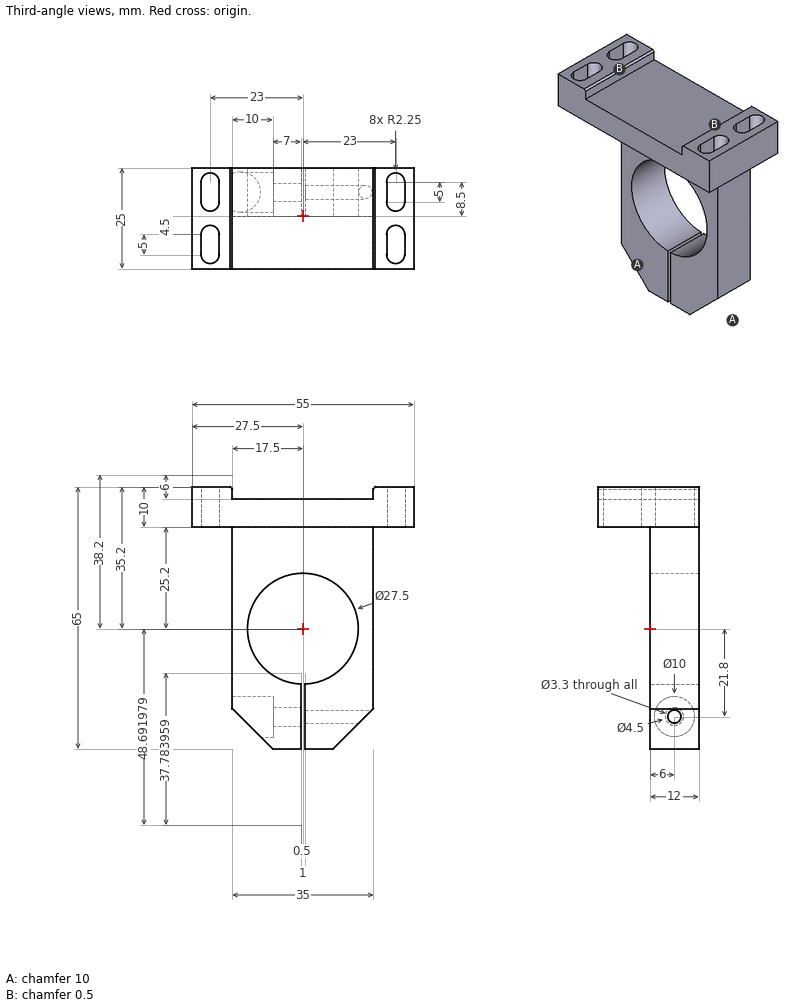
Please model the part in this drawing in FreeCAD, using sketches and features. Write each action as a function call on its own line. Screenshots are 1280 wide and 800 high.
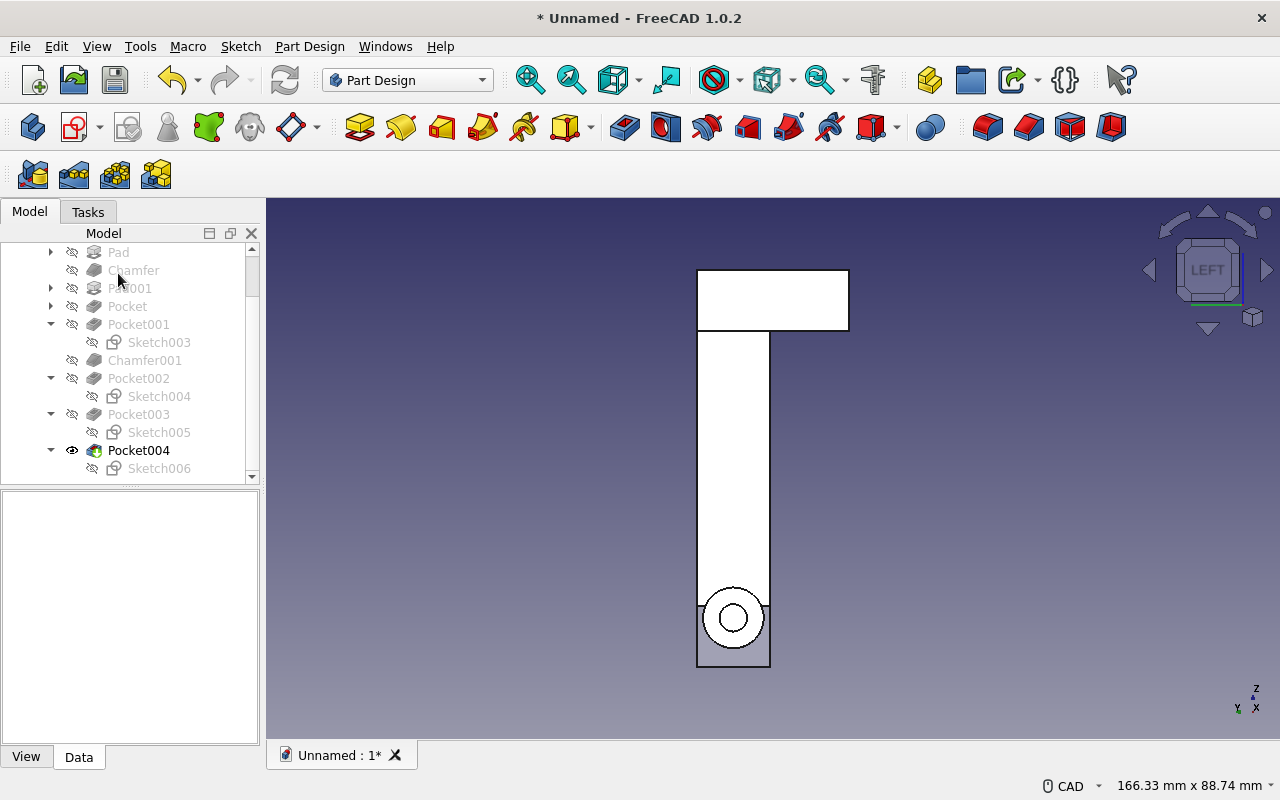
click(733, 617)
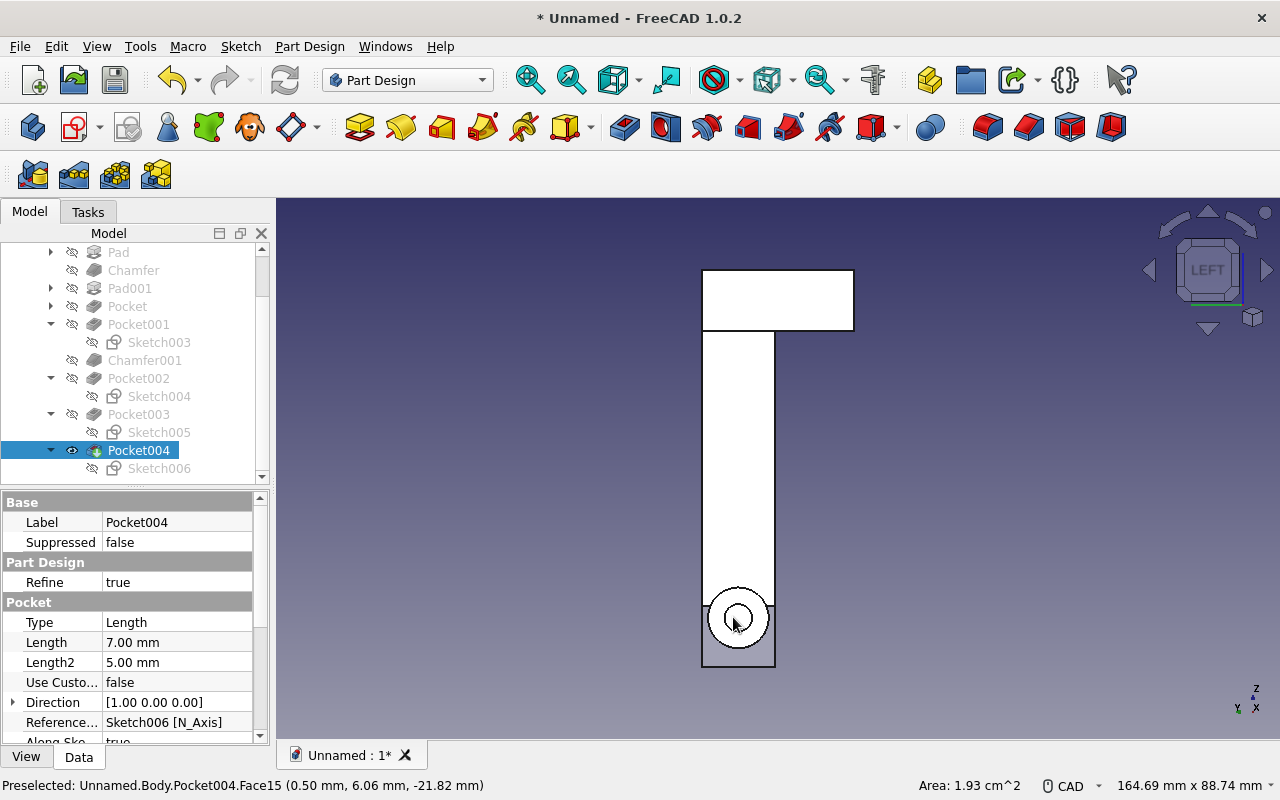
click(74, 128)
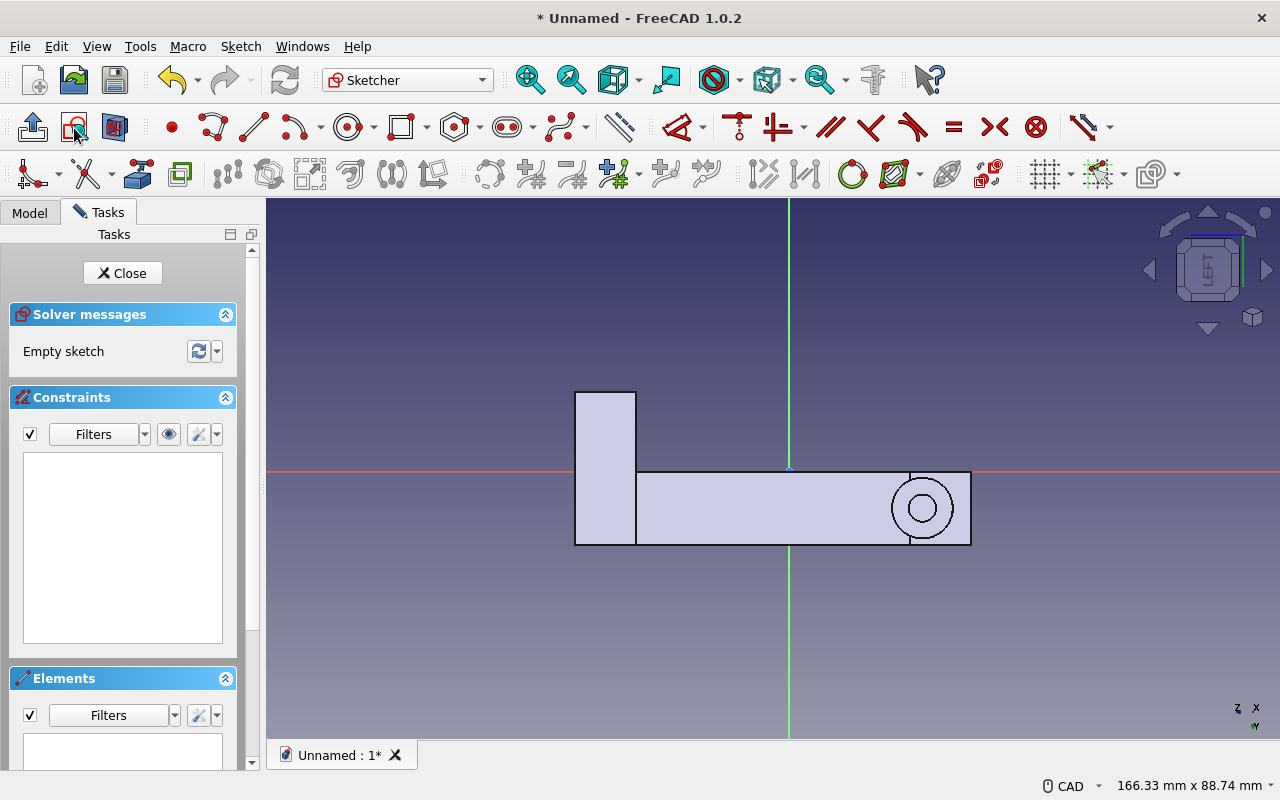
scroll(936, 511, up, 14)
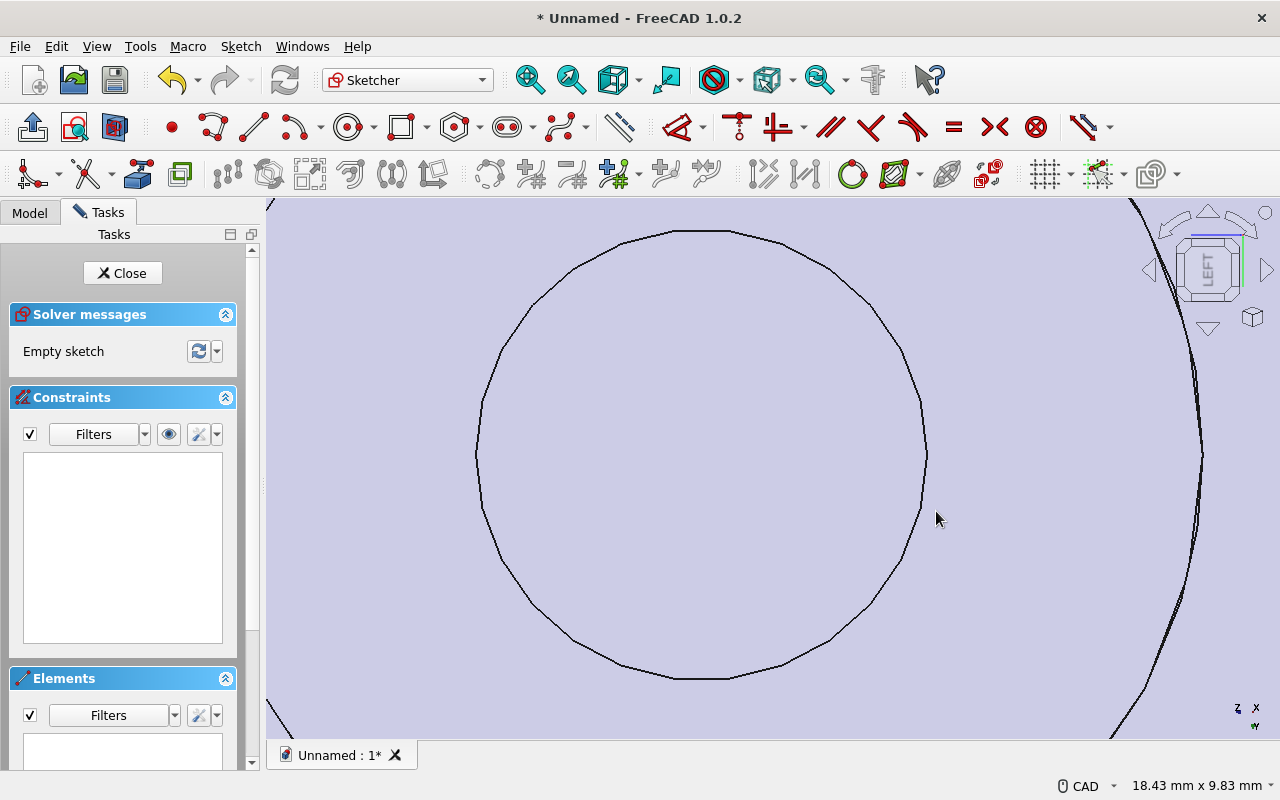
click(348, 128)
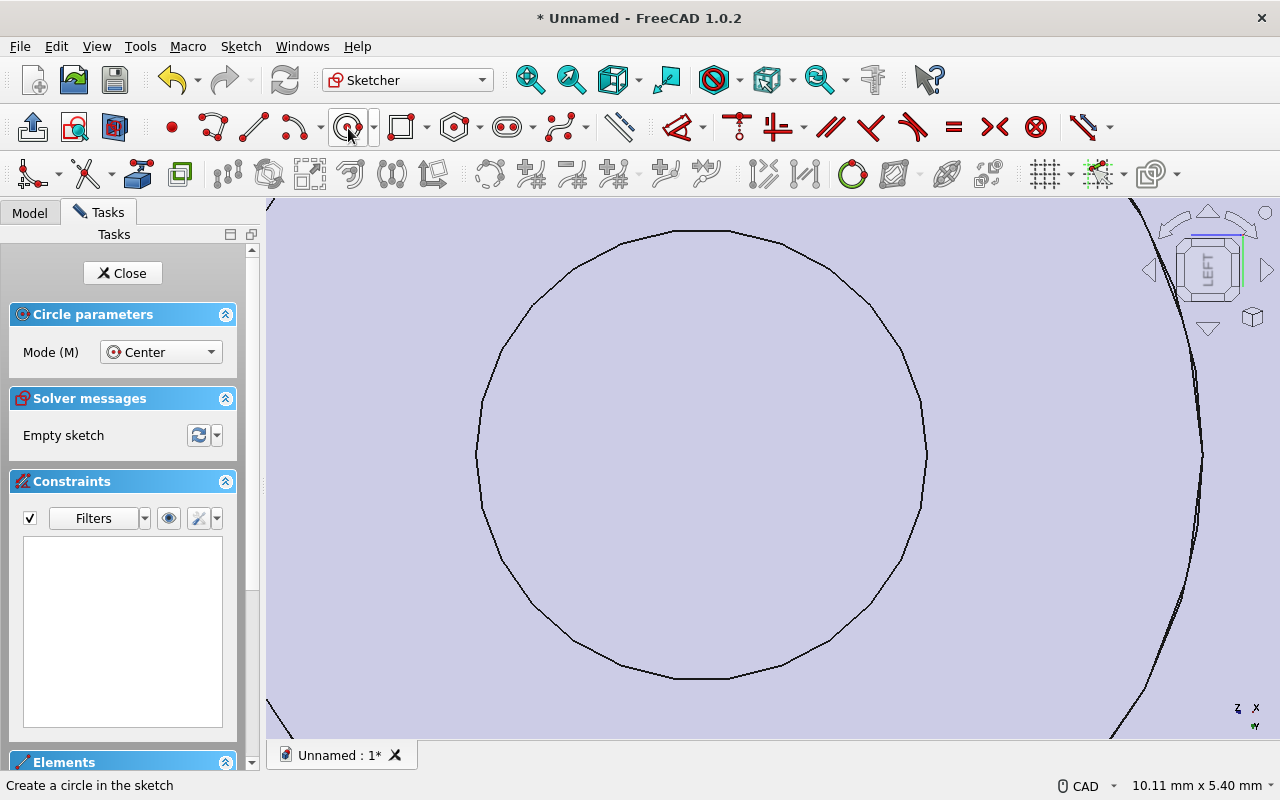
click(702, 455)
click(818, 338)
key(Escape)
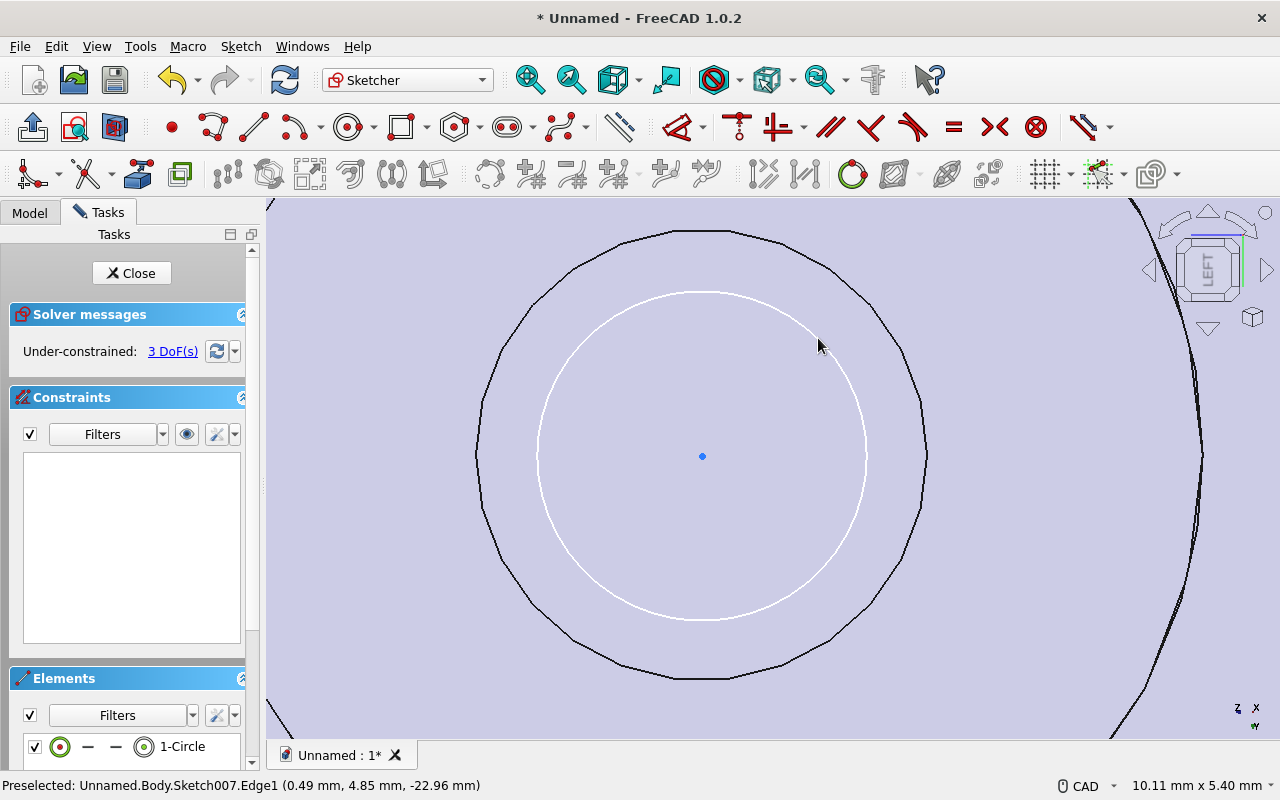
click(676, 128)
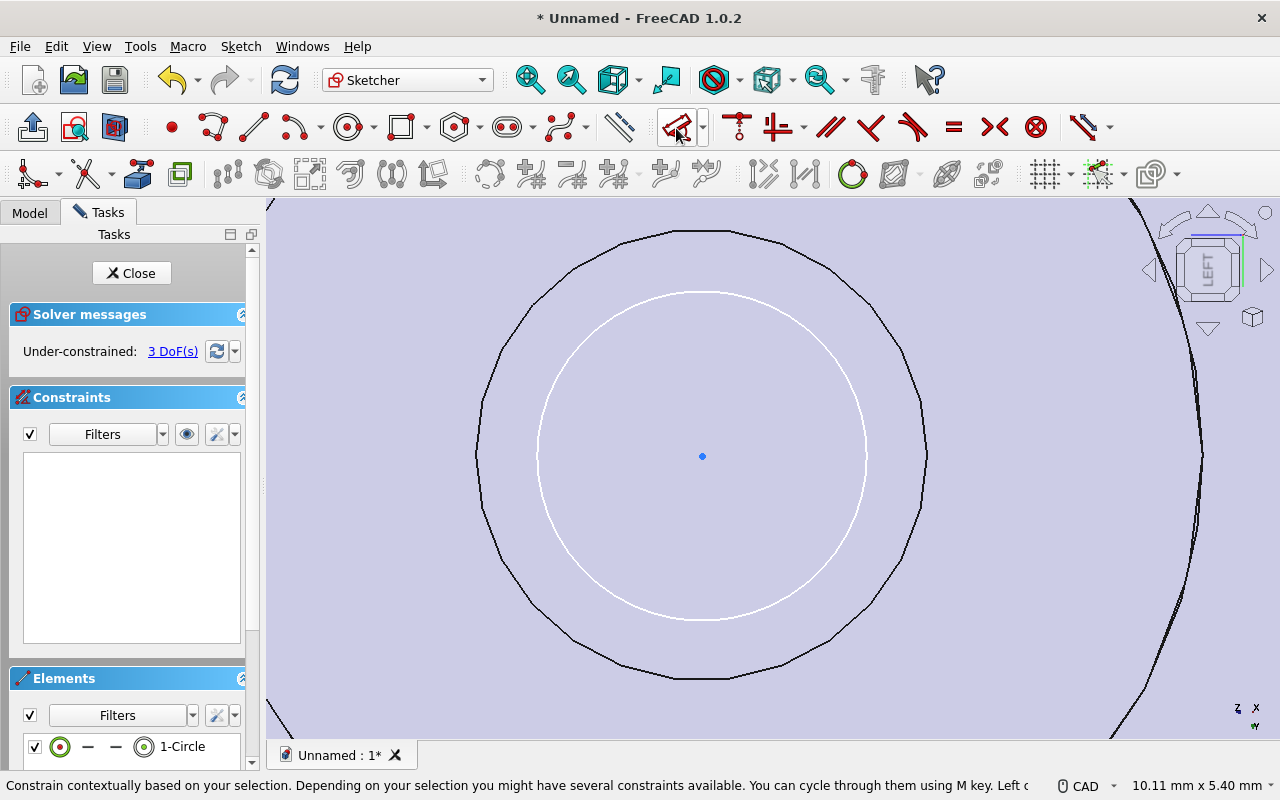
click(818, 339)
click(841, 316)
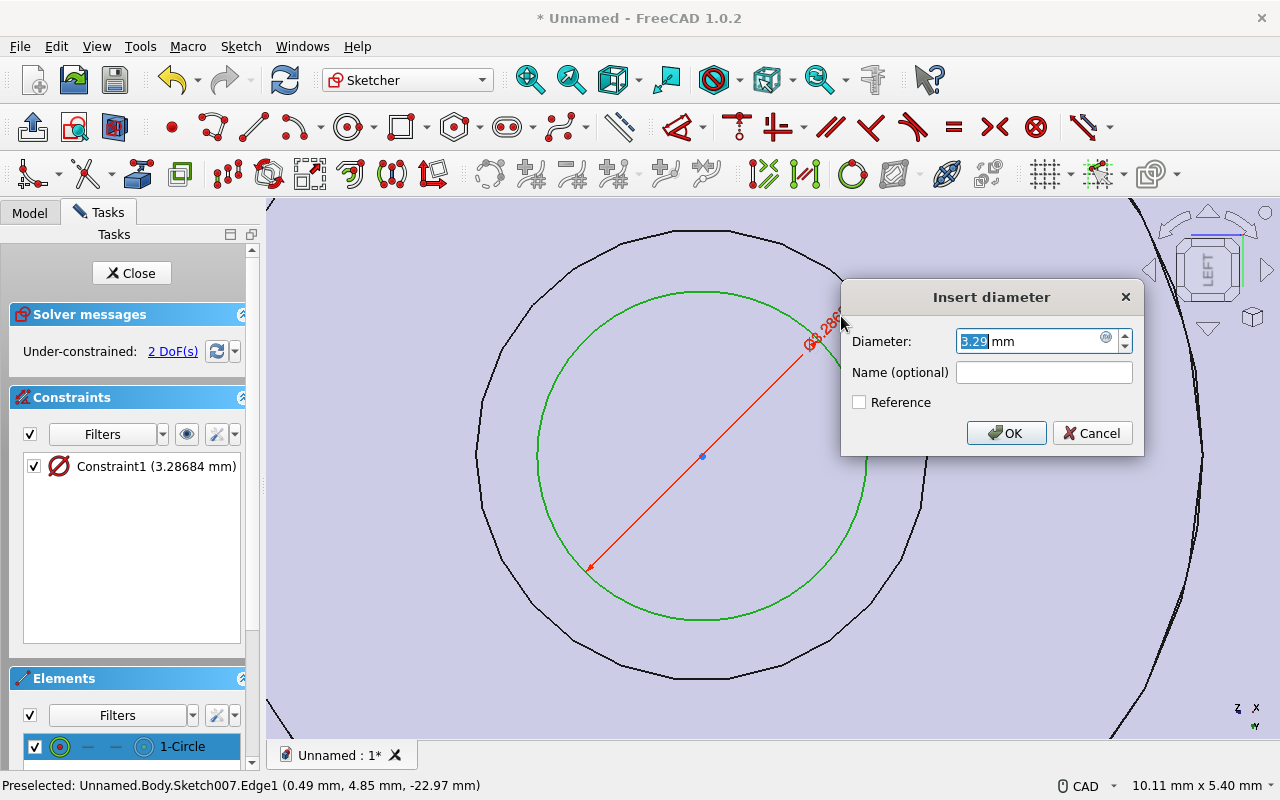
text(3.3)
key(Return)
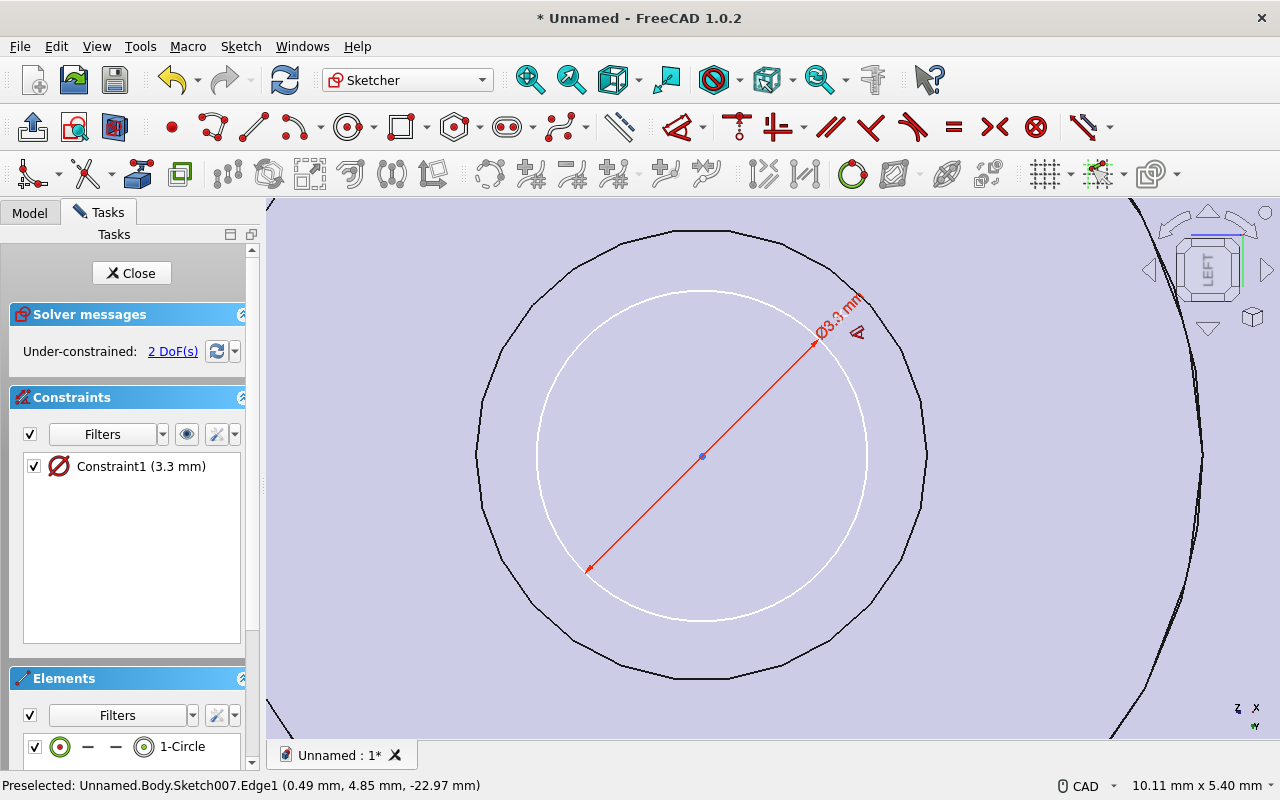
click(702, 456)
click(736, 341)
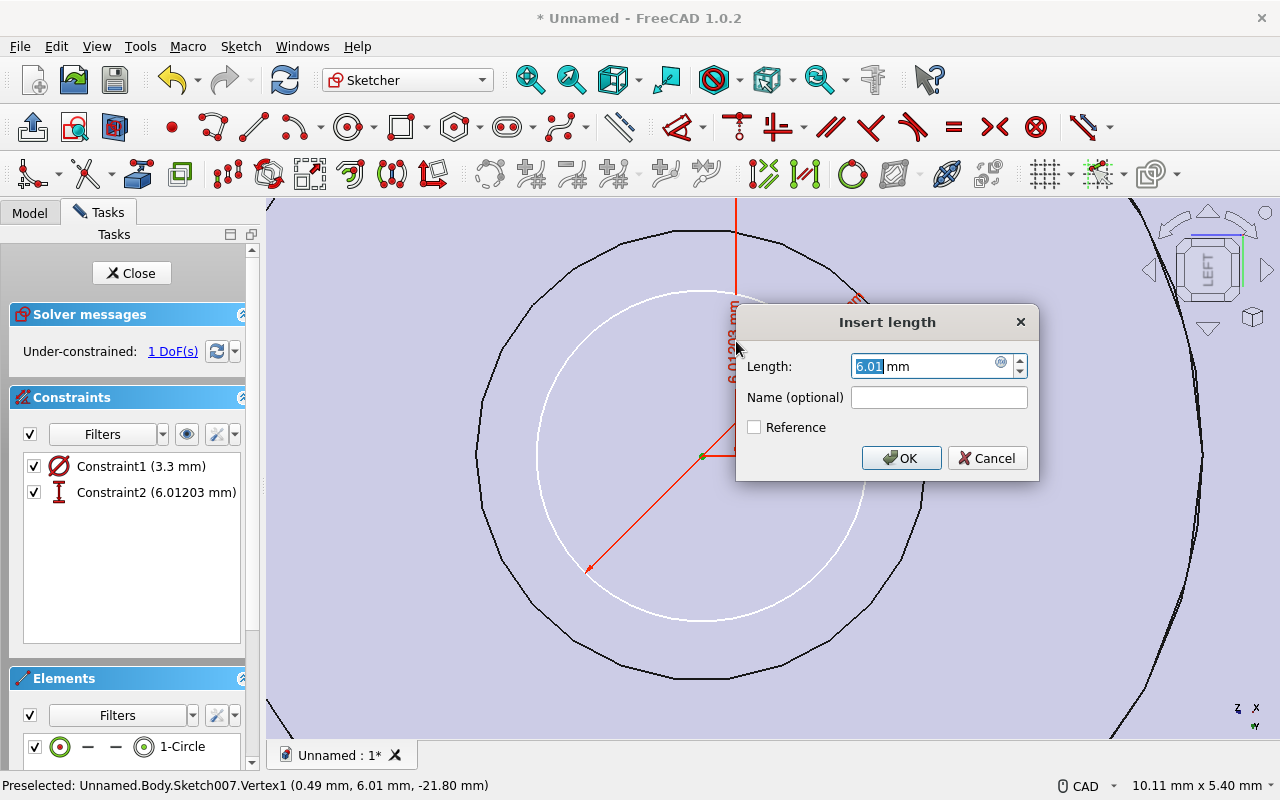
text(6)
key(Return)